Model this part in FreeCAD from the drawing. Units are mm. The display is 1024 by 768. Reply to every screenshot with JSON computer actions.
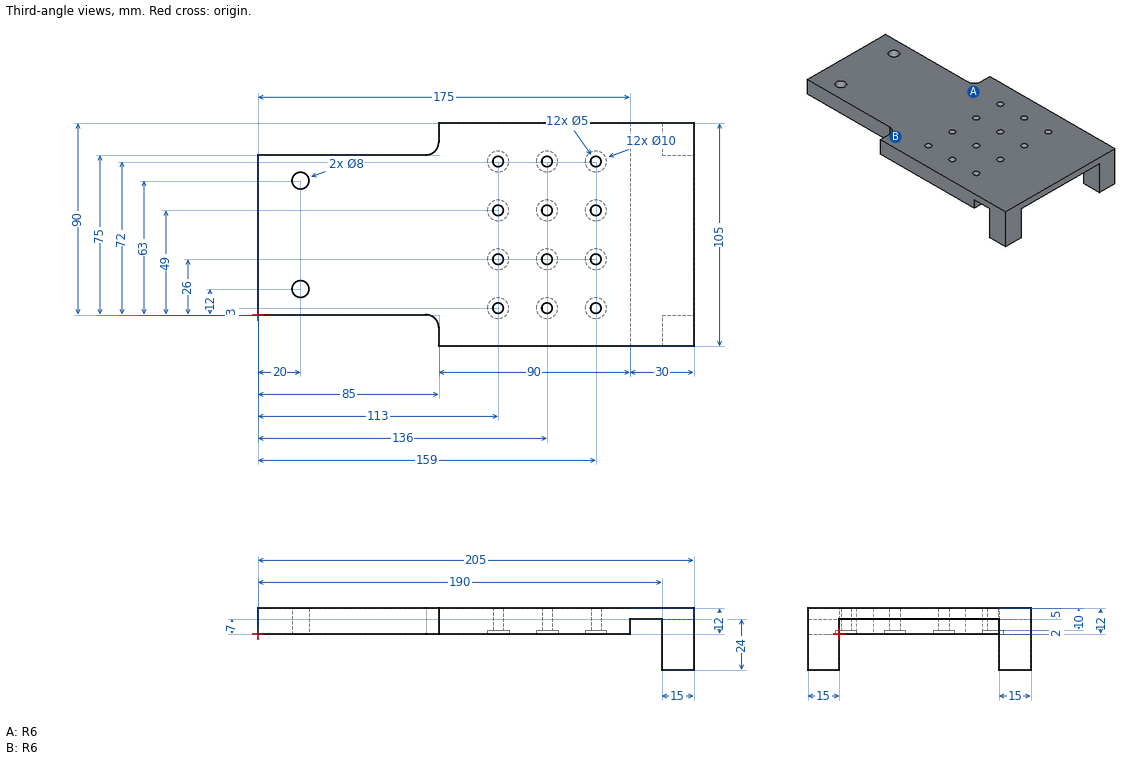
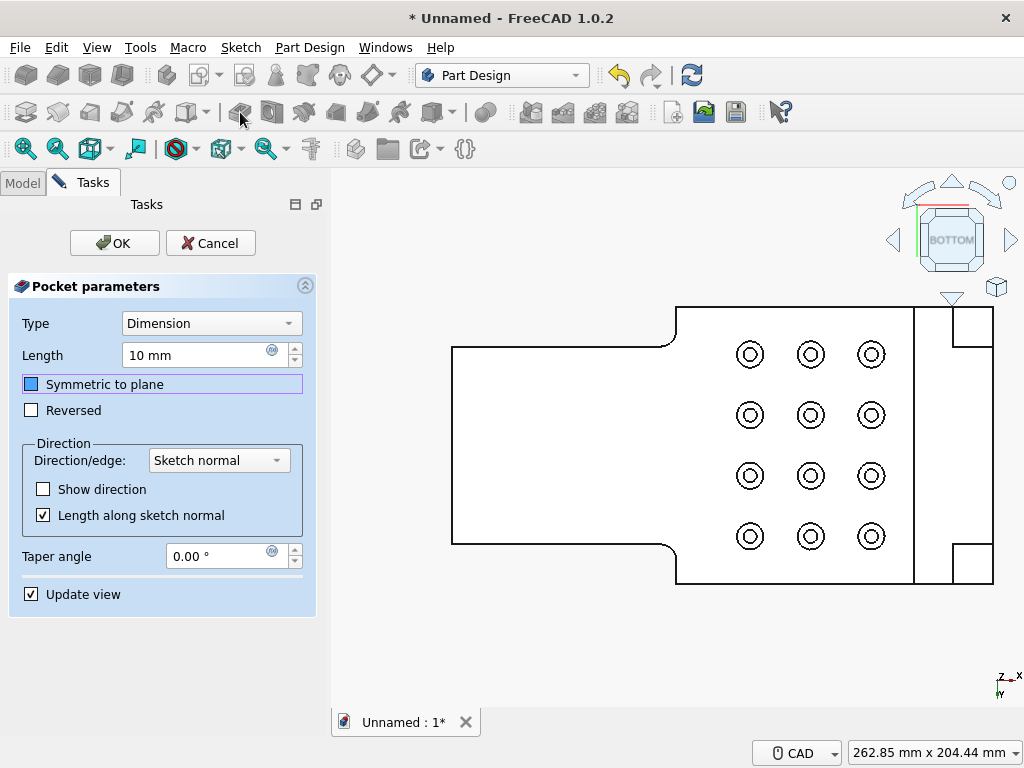
{"action": "left_click", "coordinate": [115, 243]}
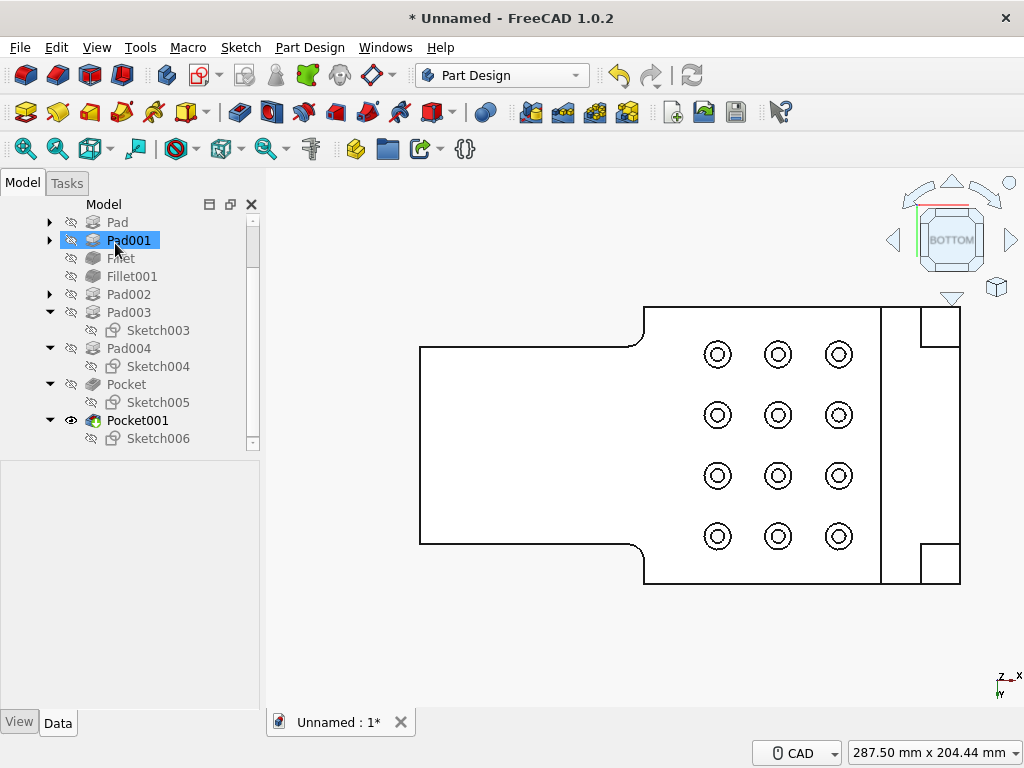
{"action": "left_click", "coordinate": [200, 76]}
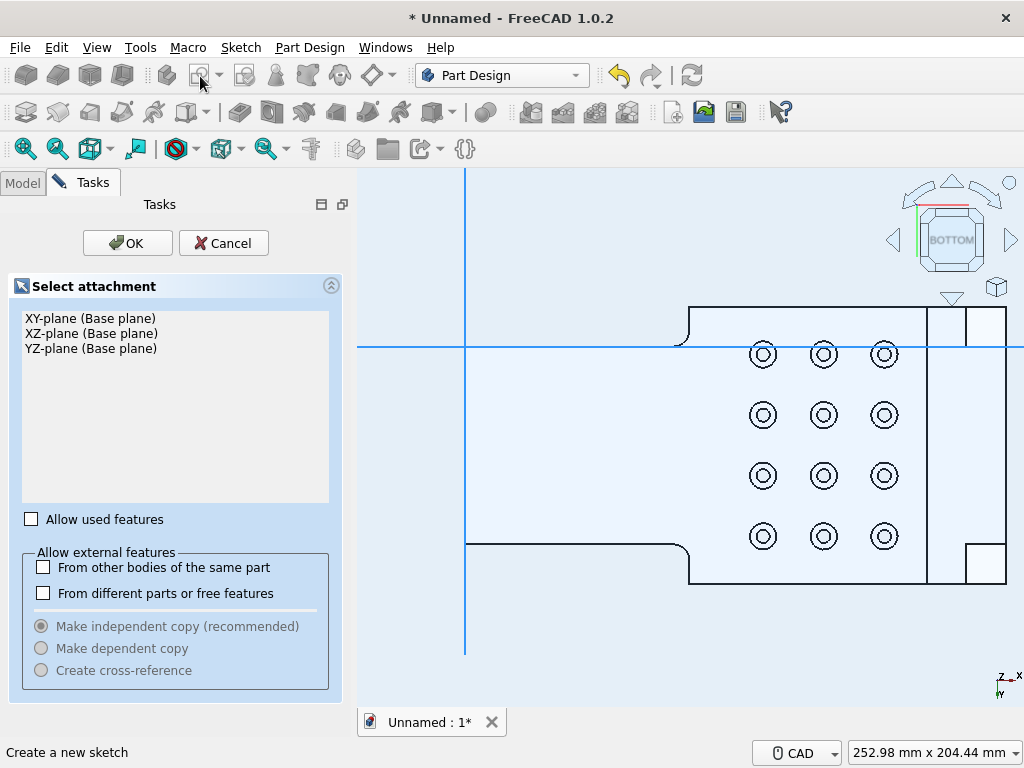
{"action": "left_click", "coordinate": [82, 318]}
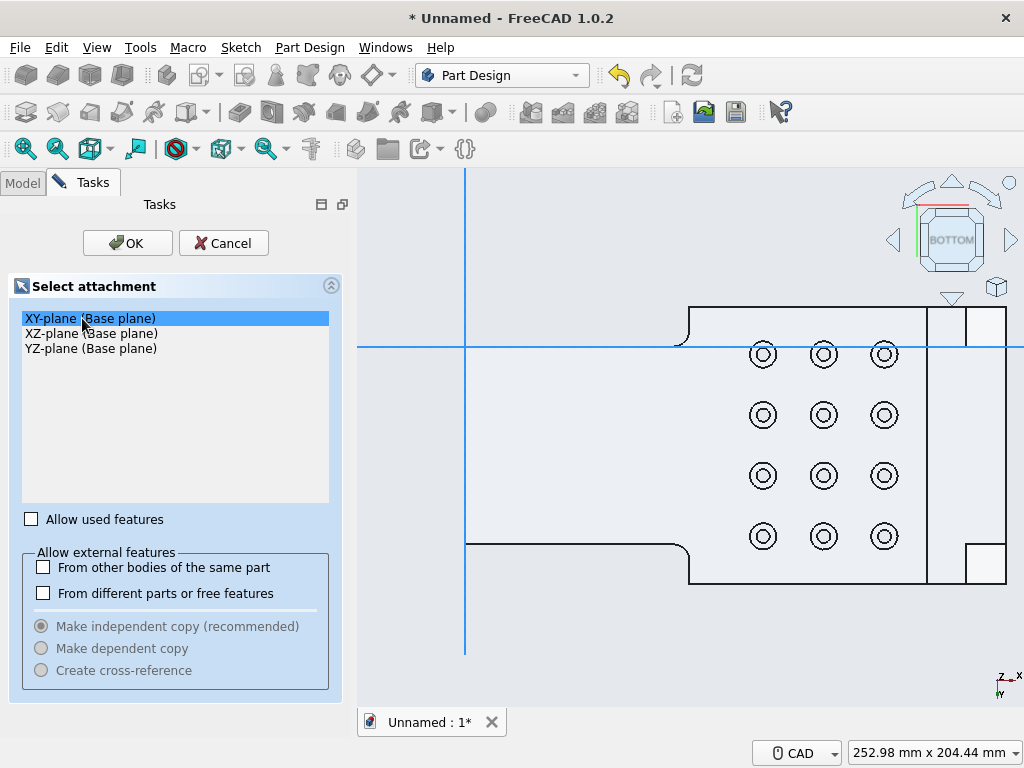
{"action": "left_click", "coordinate": [128, 243]}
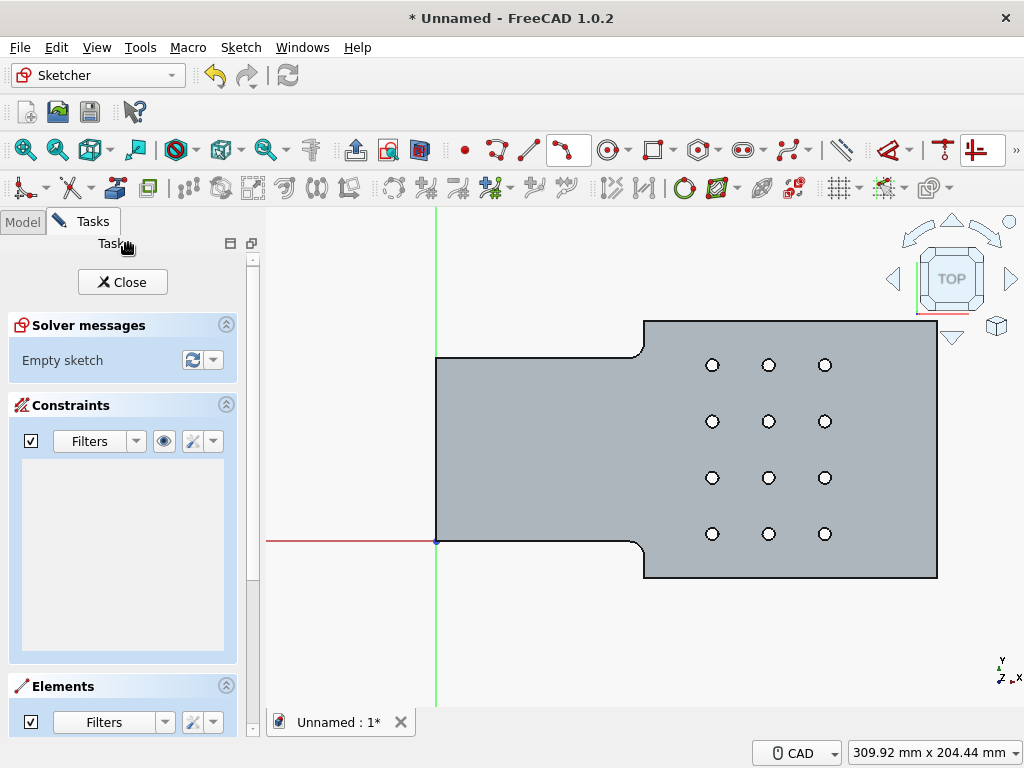
{"action": "left_click", "coordinate": [420, 150]}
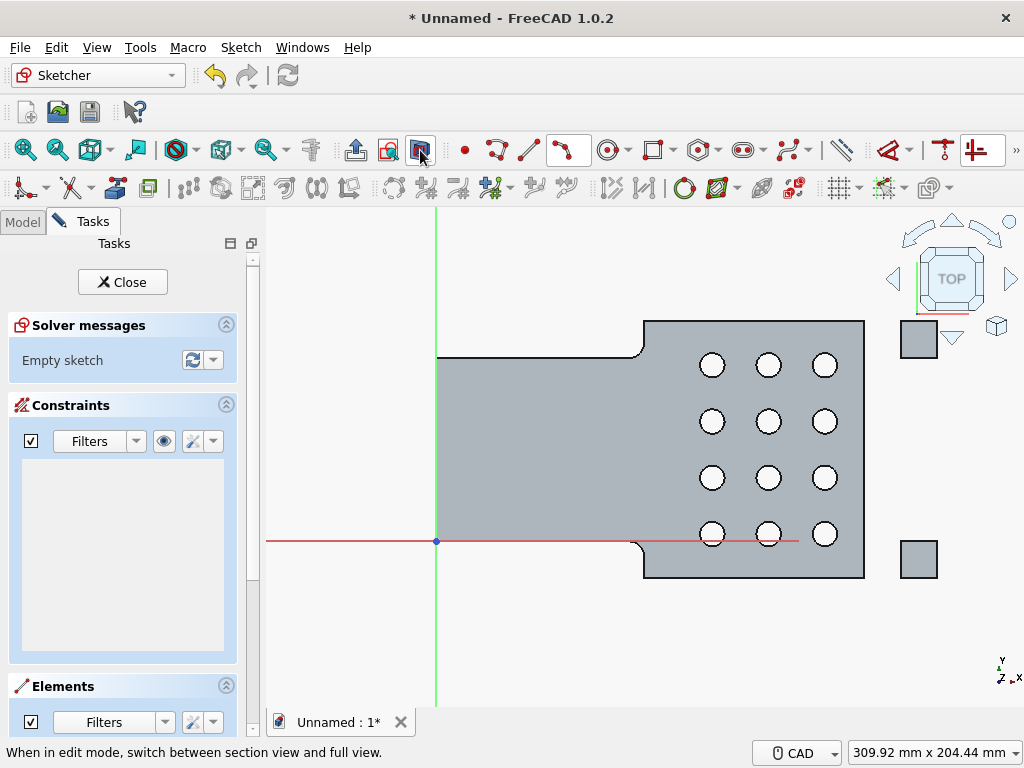
{"action": "scroll", "coordinate": [330, 462], "scroll_direction": "up", "scroll_amount": 3}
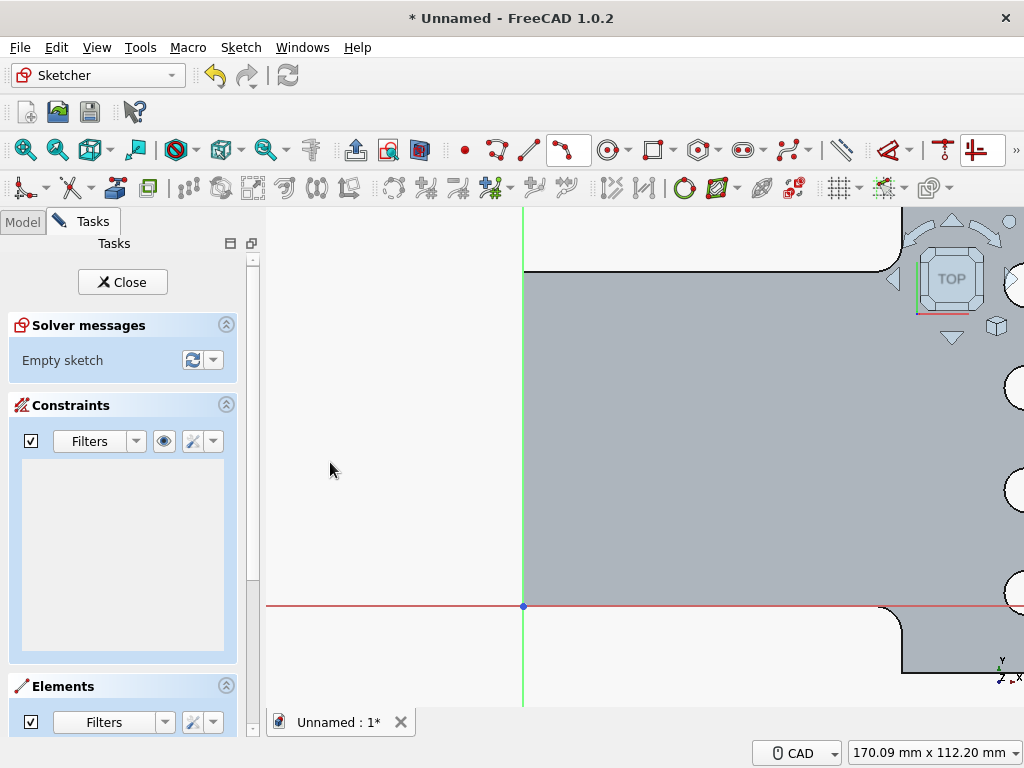
{"action": "left_click", "coordinate": [608, 150]}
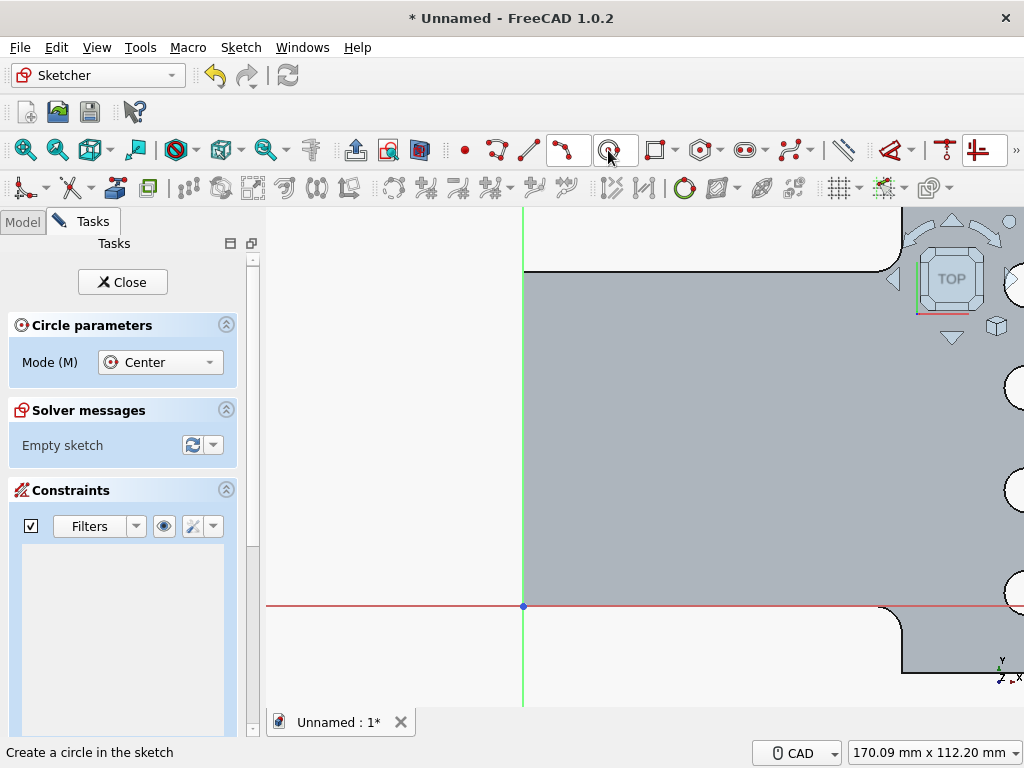
{"action": "scroll", "coordinate": [612, 325], "scroll_direction": "up", "scroll_amount": 2}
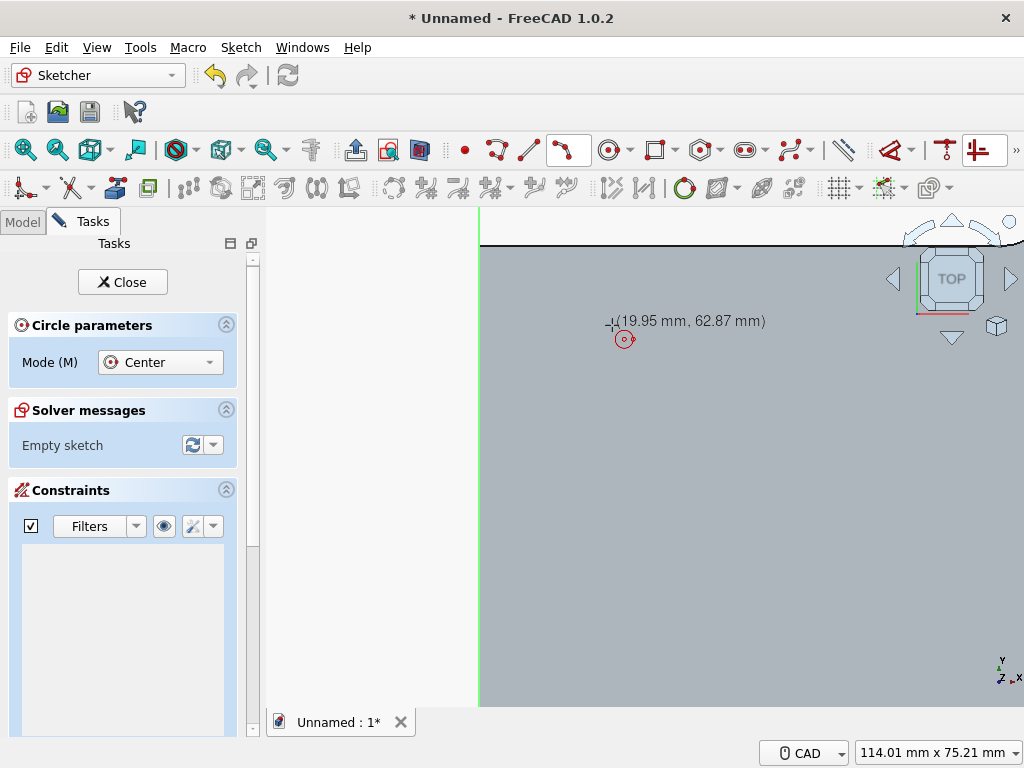
{"action": "left_click", "coordinate": [612, 326]}
{"action": "mouse_move", "coordinate": [631, 307]}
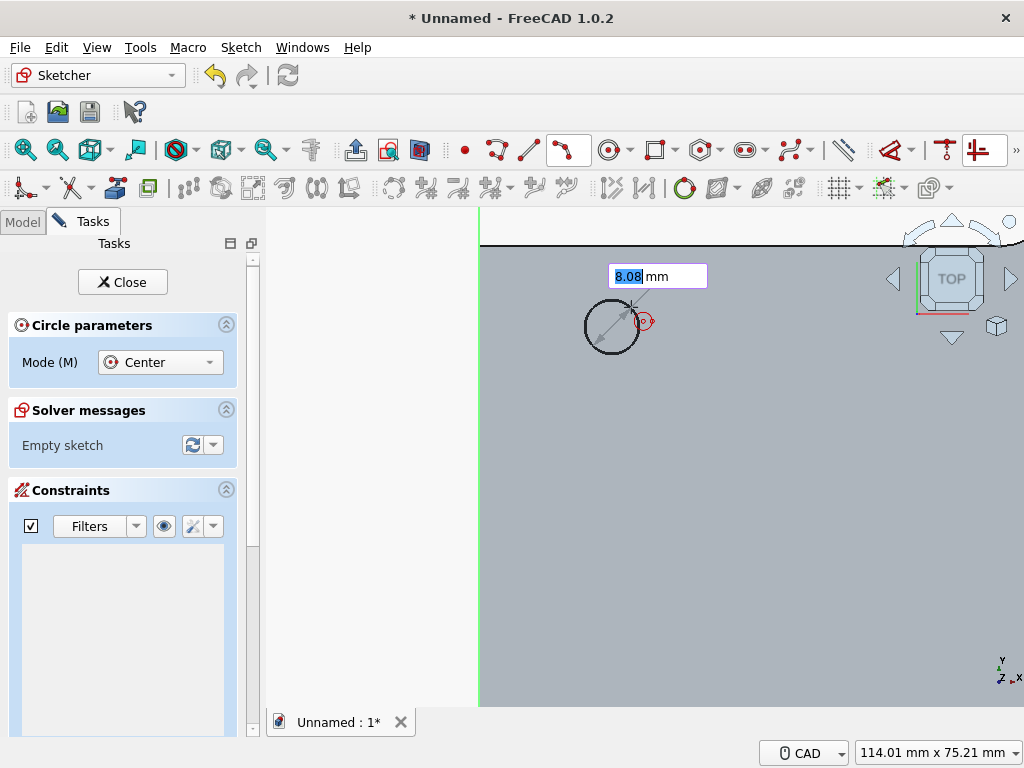
{"action": "type", "text": "8"}
{"action": "key", "text": "Return"}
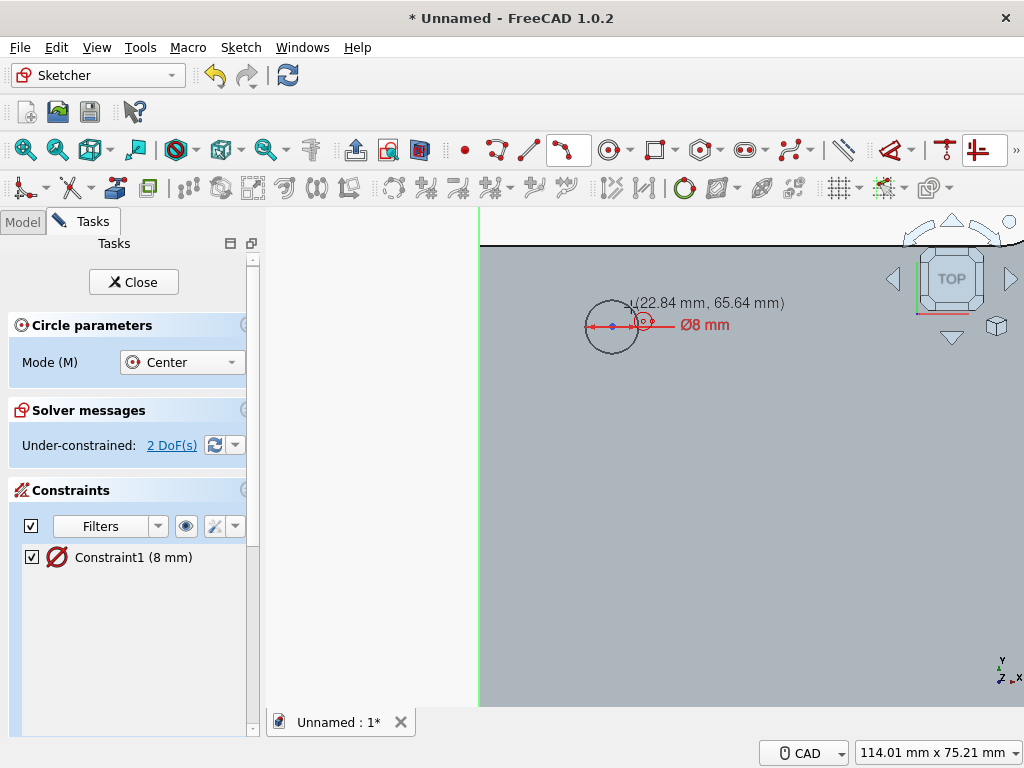
{"action": "left_click", "coordinate": [612, 665]}
{"action": "mouse_move", "coordinate": [631, 646]}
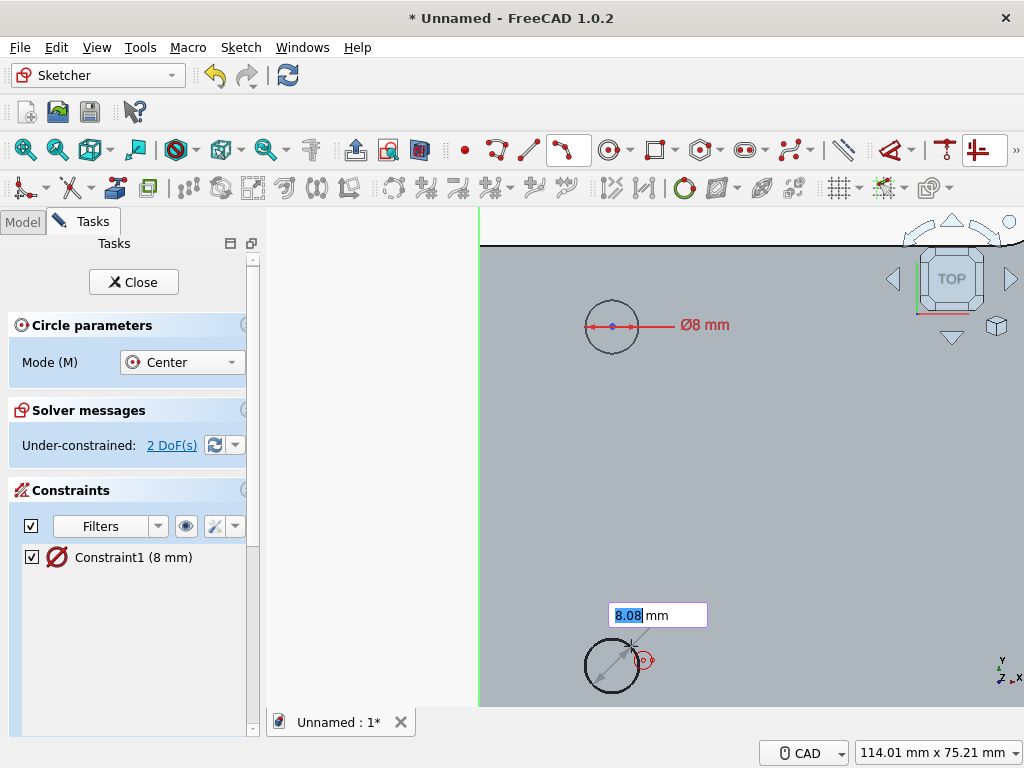
{"action": "type", "text": "8"}
{"action": "key", "text": "Return"}
{"action": "key", "text": "Escape"}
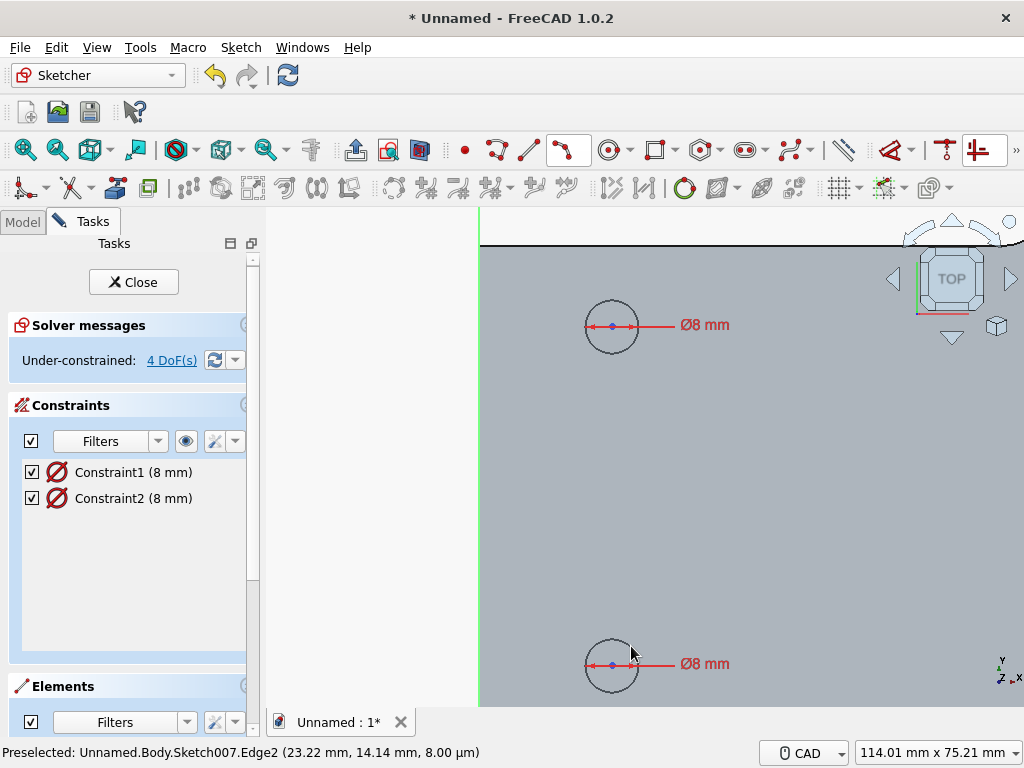
{"action": "left_click", "coordinate": [612, 327]}